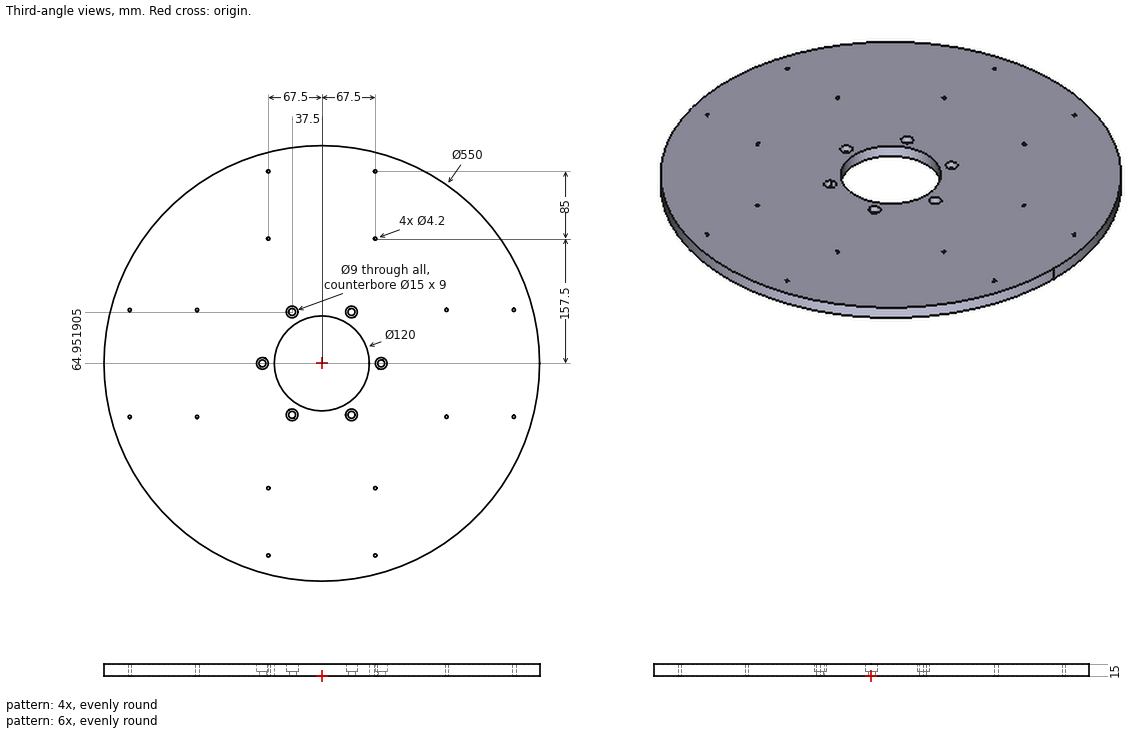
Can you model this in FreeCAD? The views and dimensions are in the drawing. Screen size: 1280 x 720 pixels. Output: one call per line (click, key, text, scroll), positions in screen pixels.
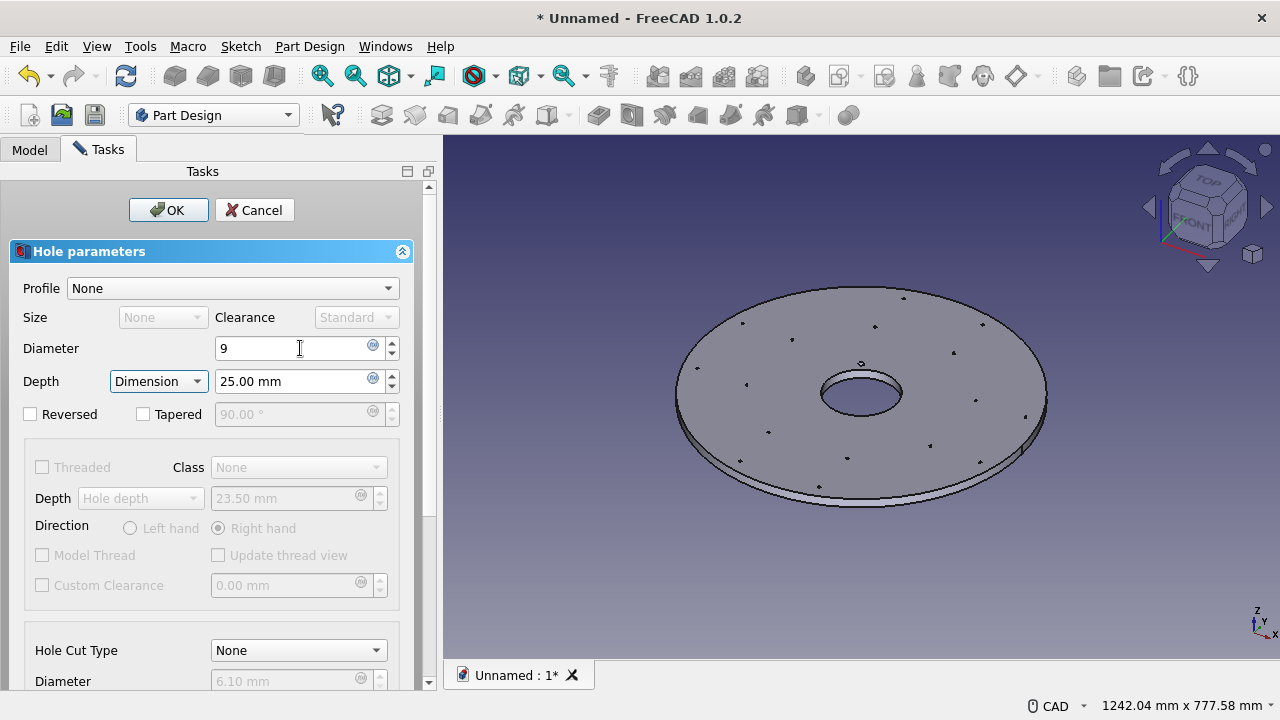
click(160, 382)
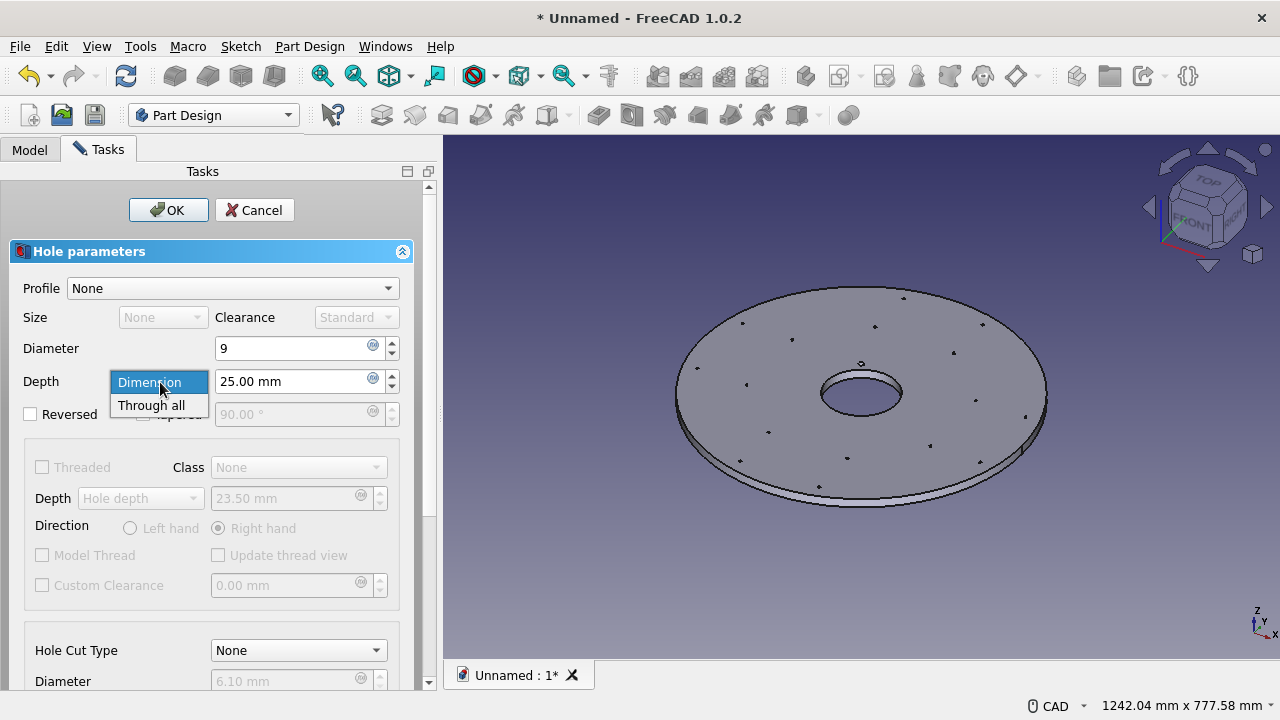
click(158, 406)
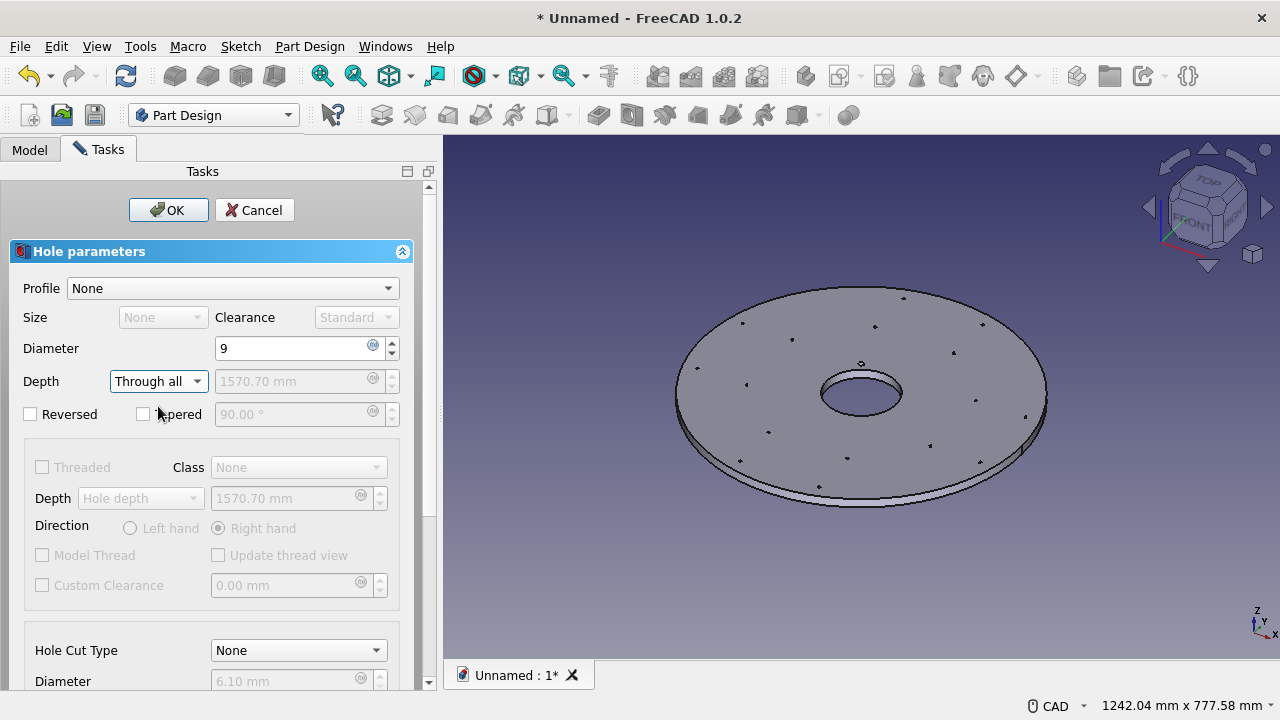
click(300, 650)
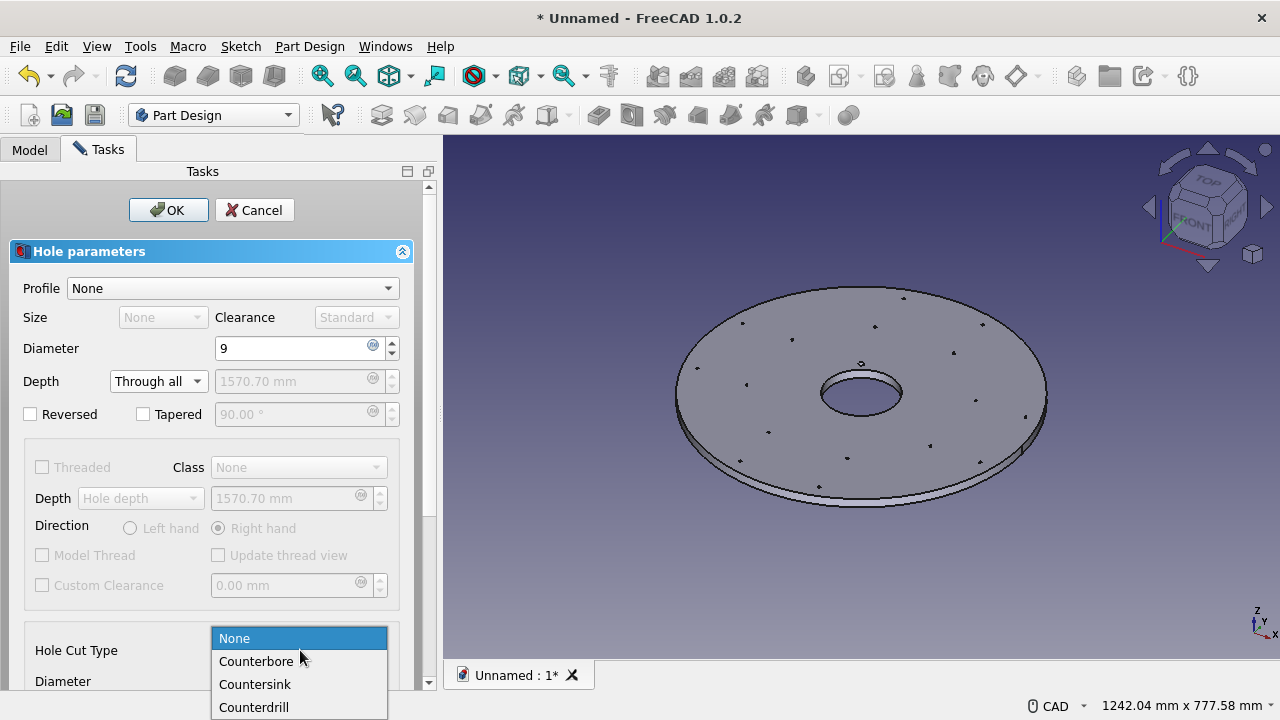
click(298, 662)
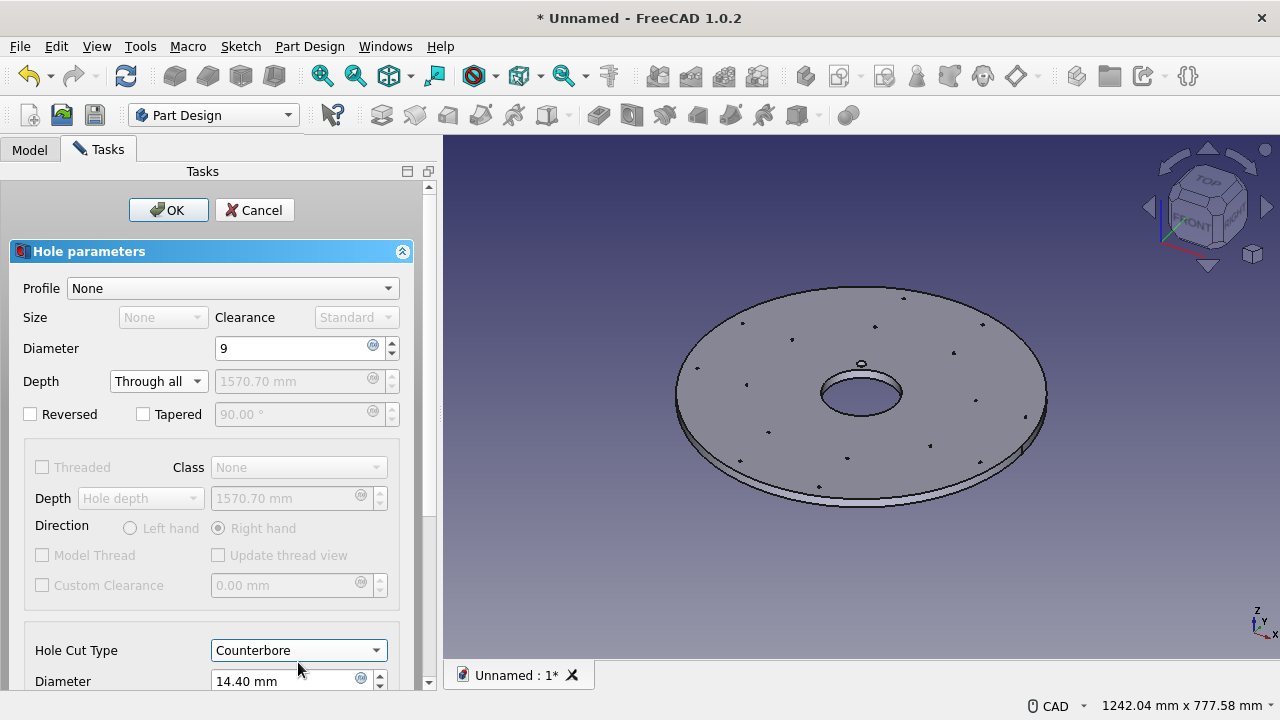
scroll(429, 436, down, 2)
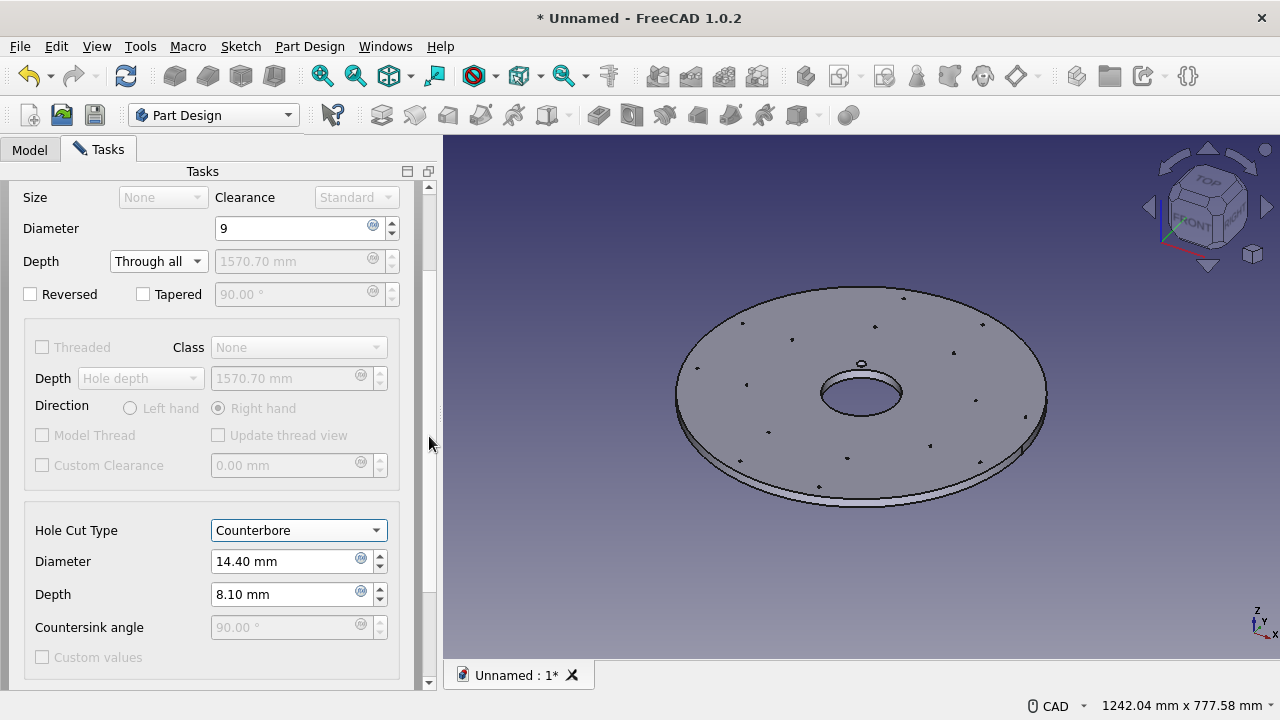
triple_click(292, 562)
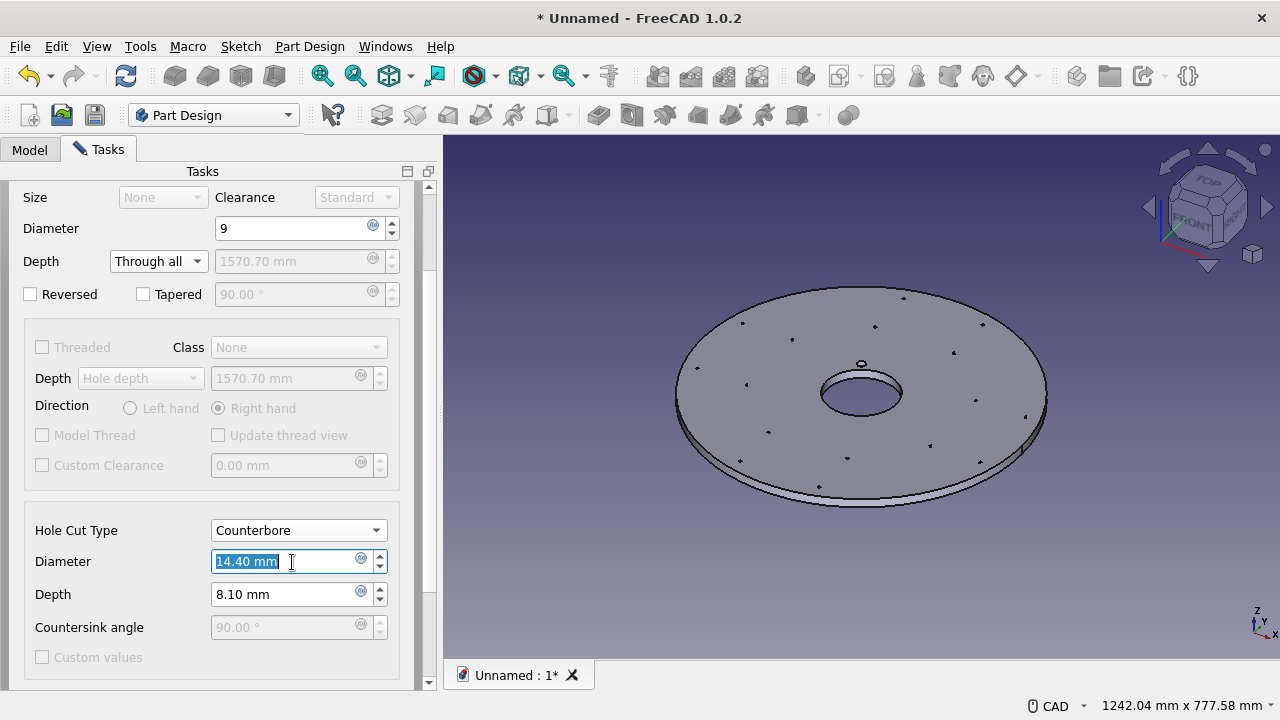
text(15)
key(Tab)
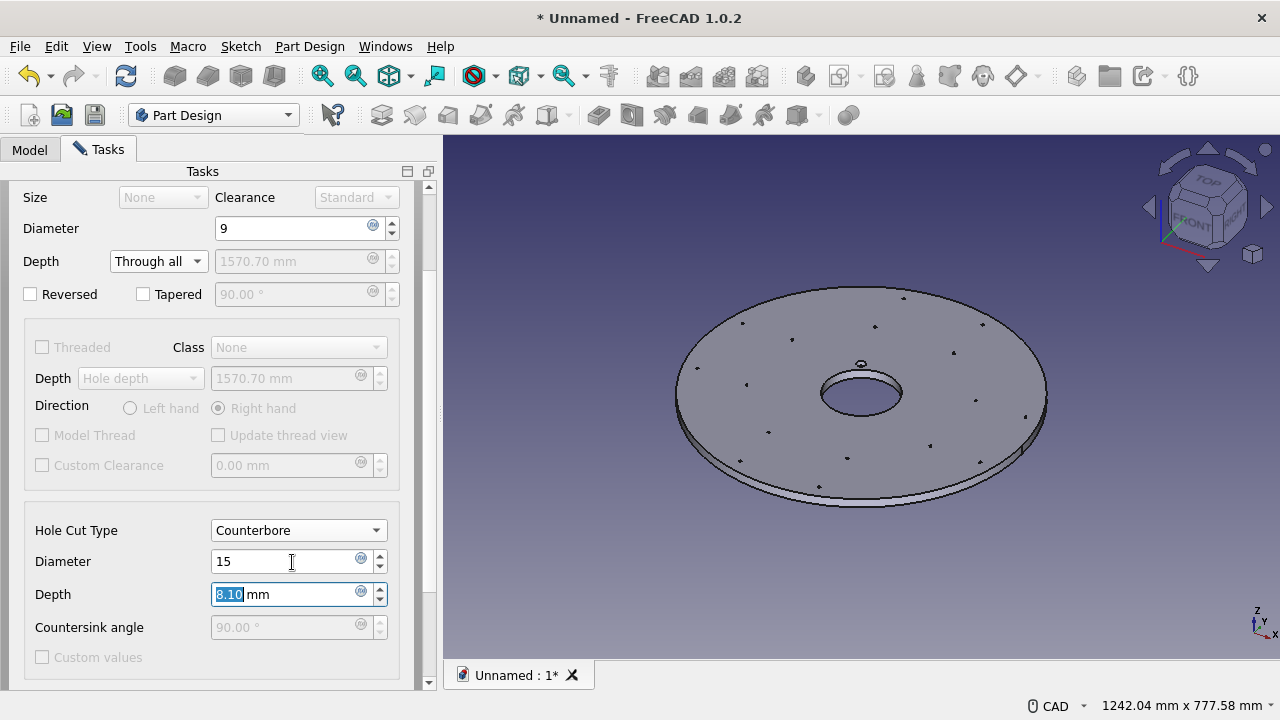
text(9)
key(Tab)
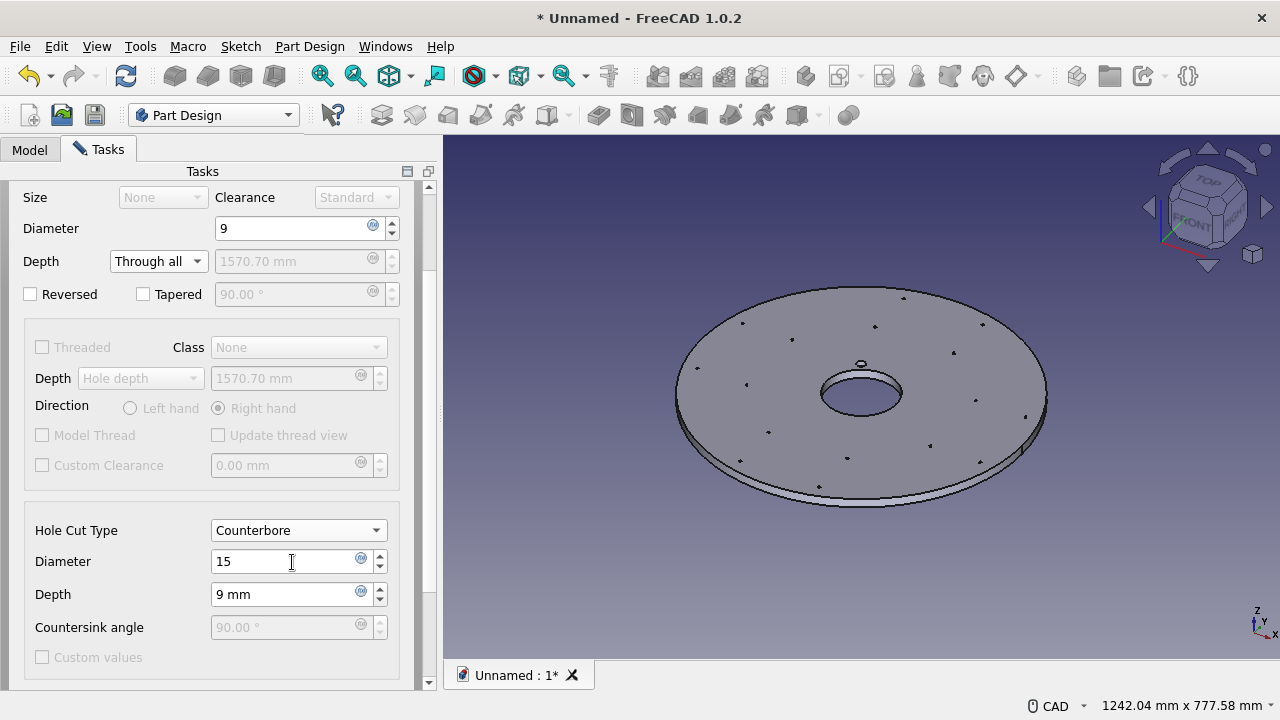
scroll(429, 436, up, 3)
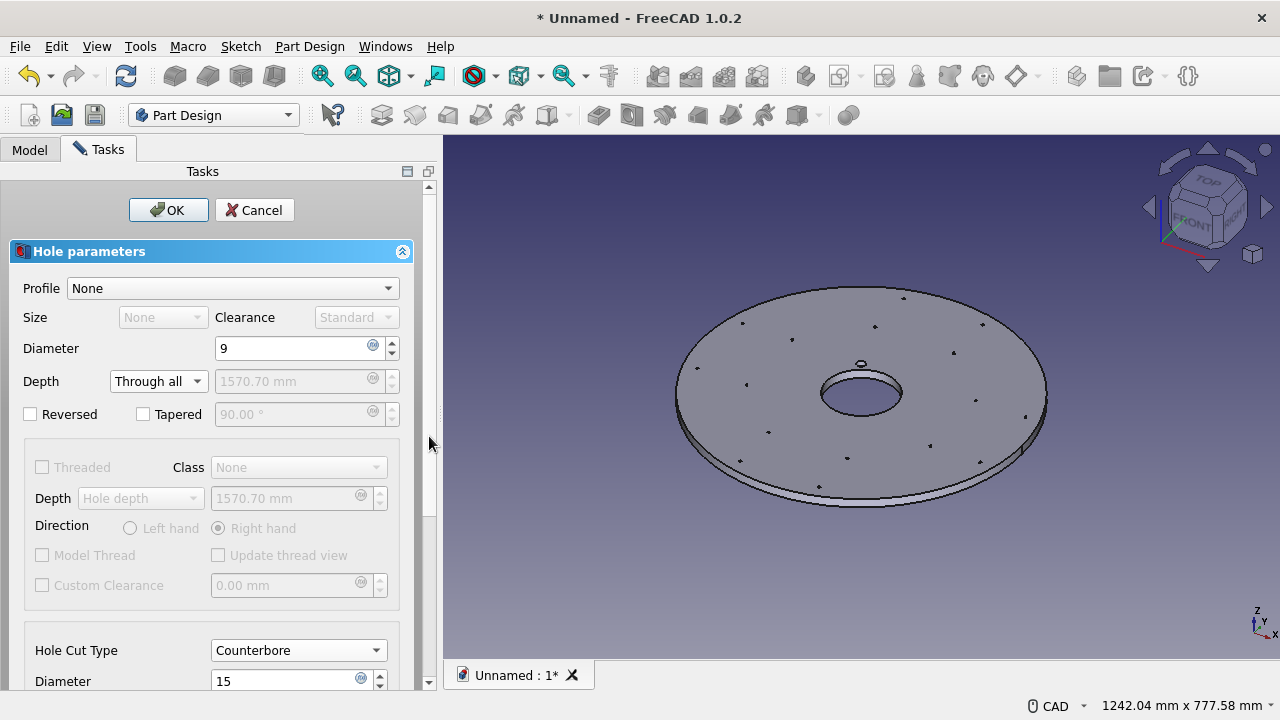
click(169, 210)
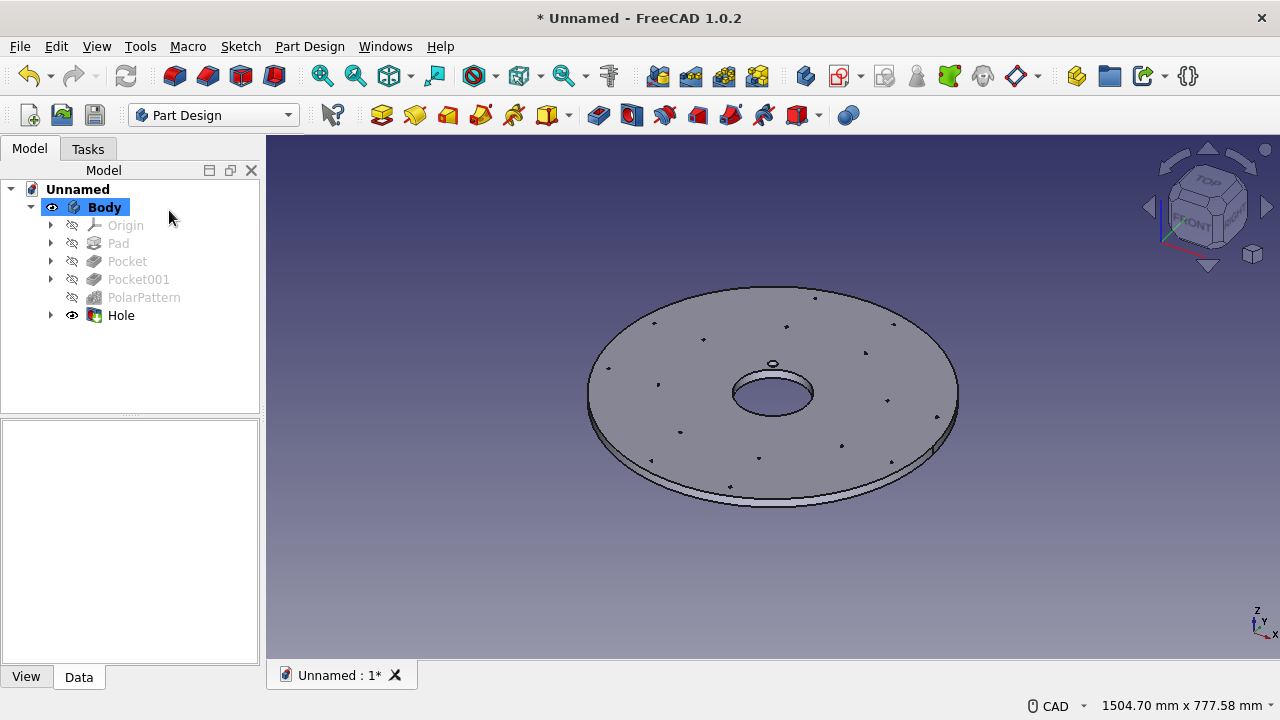
click(117, 315)